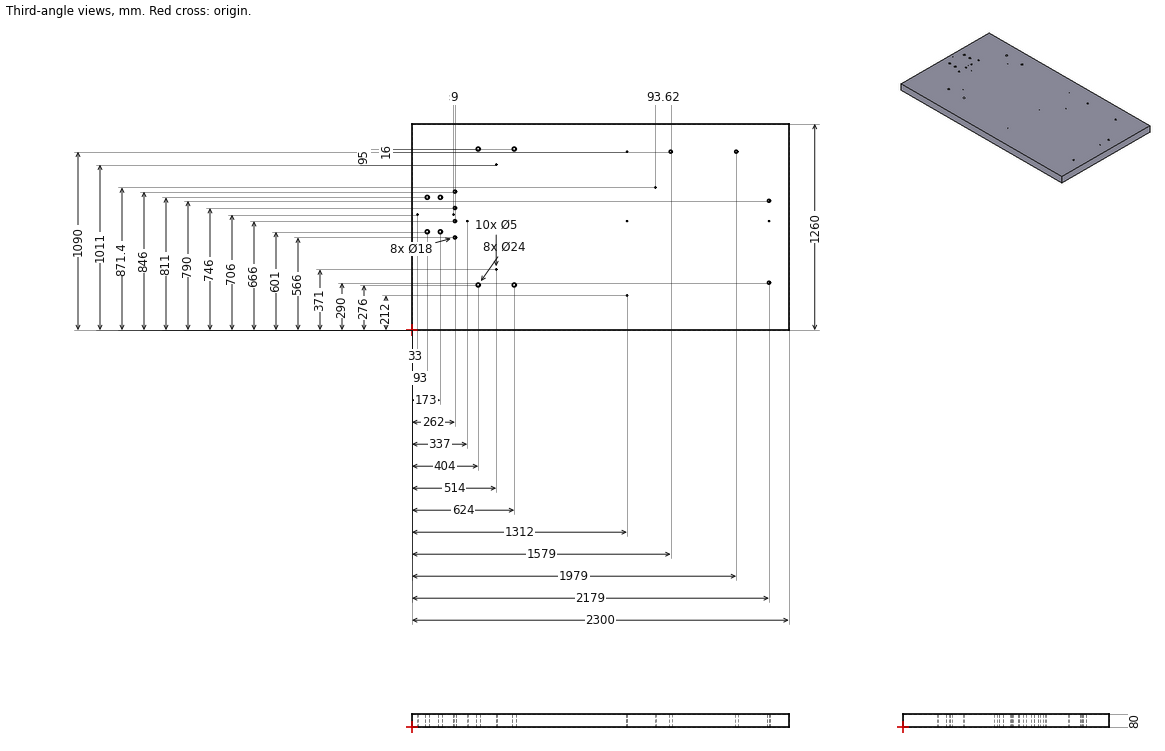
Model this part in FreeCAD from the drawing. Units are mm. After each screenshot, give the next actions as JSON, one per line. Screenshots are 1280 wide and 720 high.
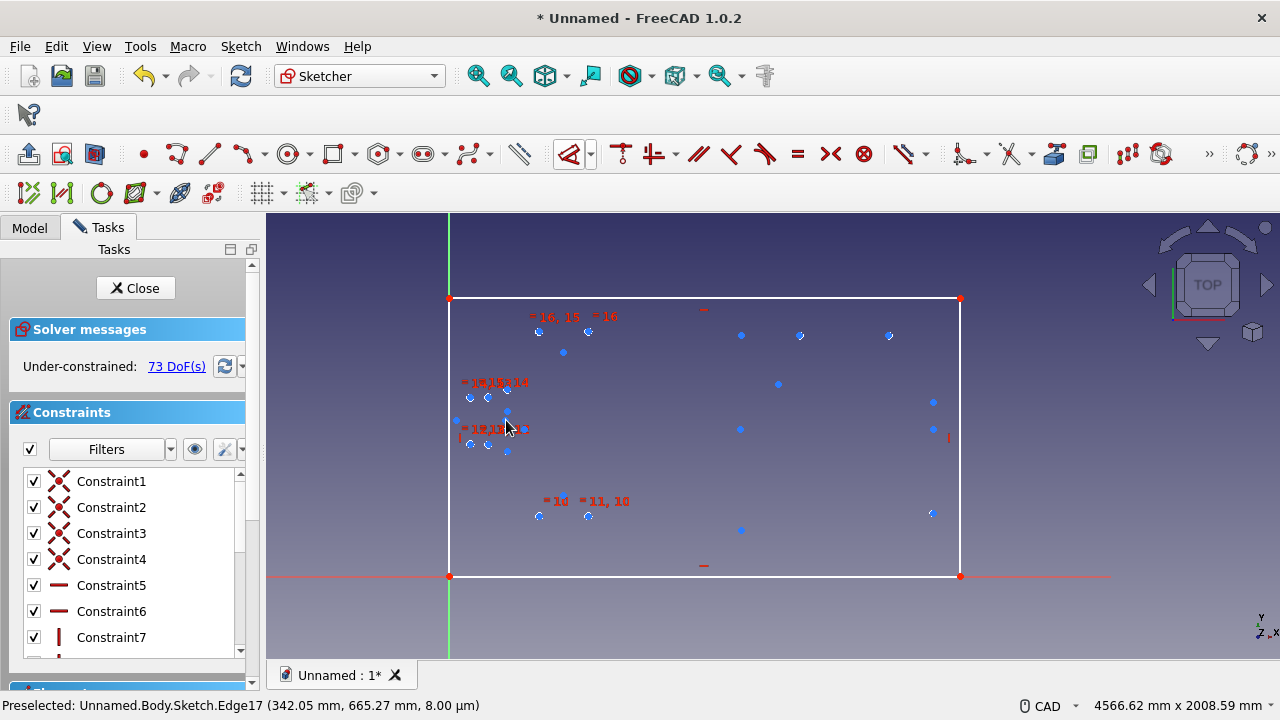
{"action": "scroll", "coordinate": [564, 352], "scroll_direction": "up", "scroll_amount": 12}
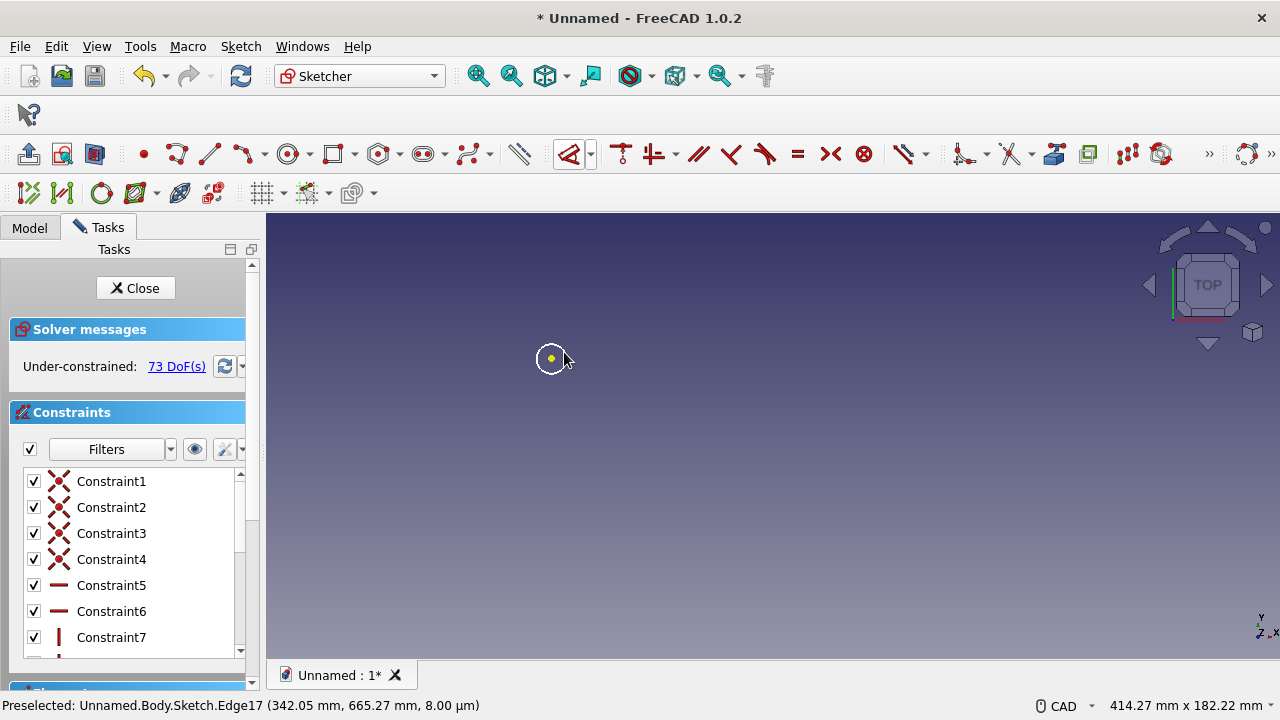
{"action": "left_click", "coordinate": [562, 349]}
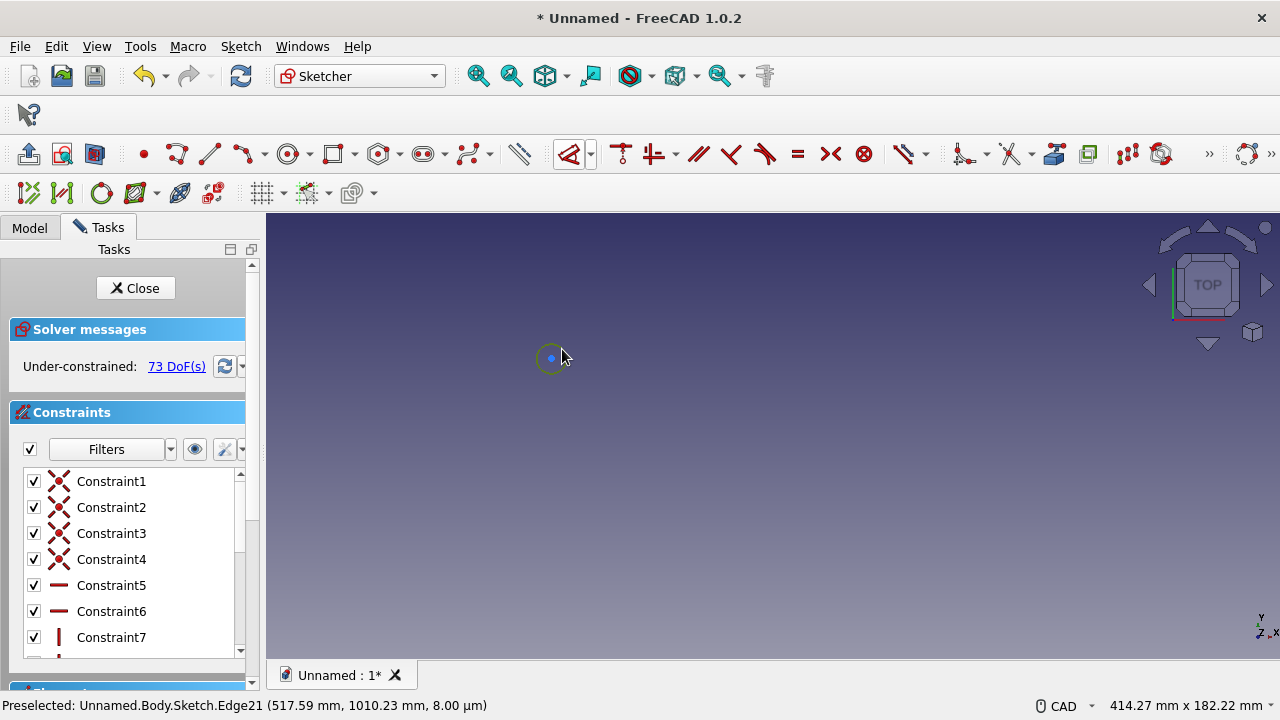
{"action": "scroll", "coordinate": [564, 351], "scroll_direction": "down", "scroll_amount": 12}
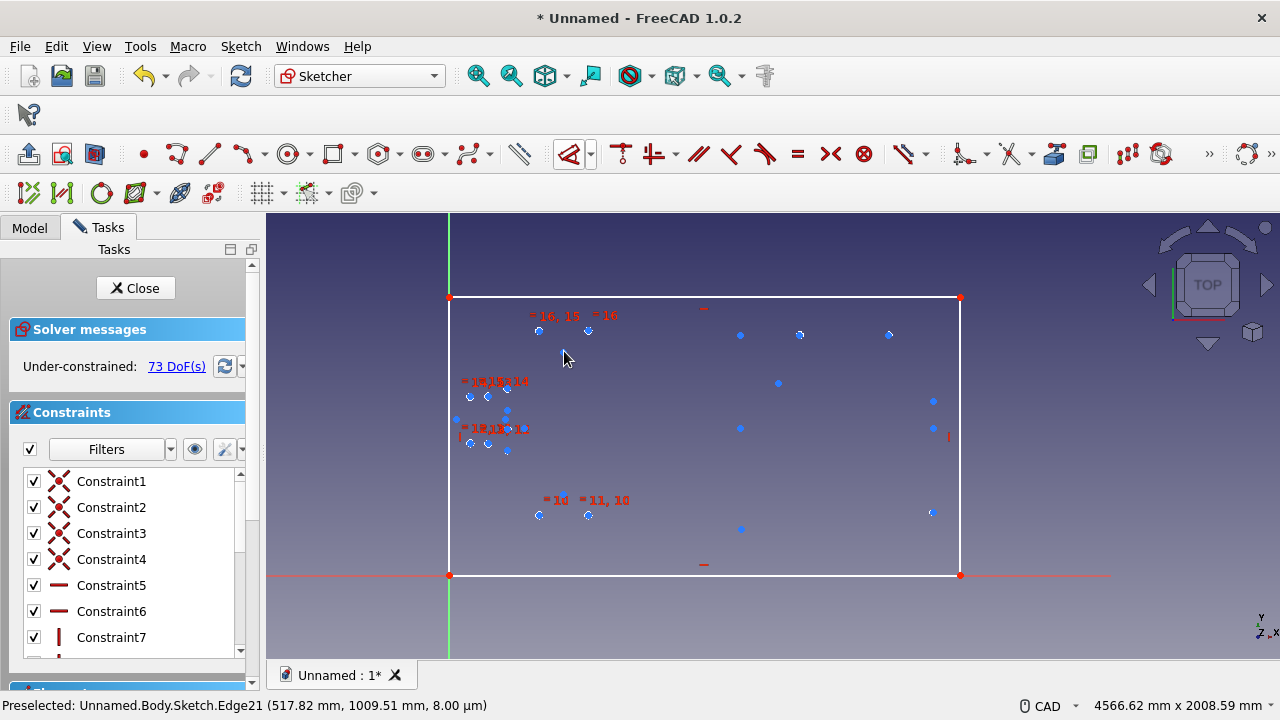
{"action": "scroll", "coordinate": [742, 428], "scroll_direction": "up", "scroll_amount": 13}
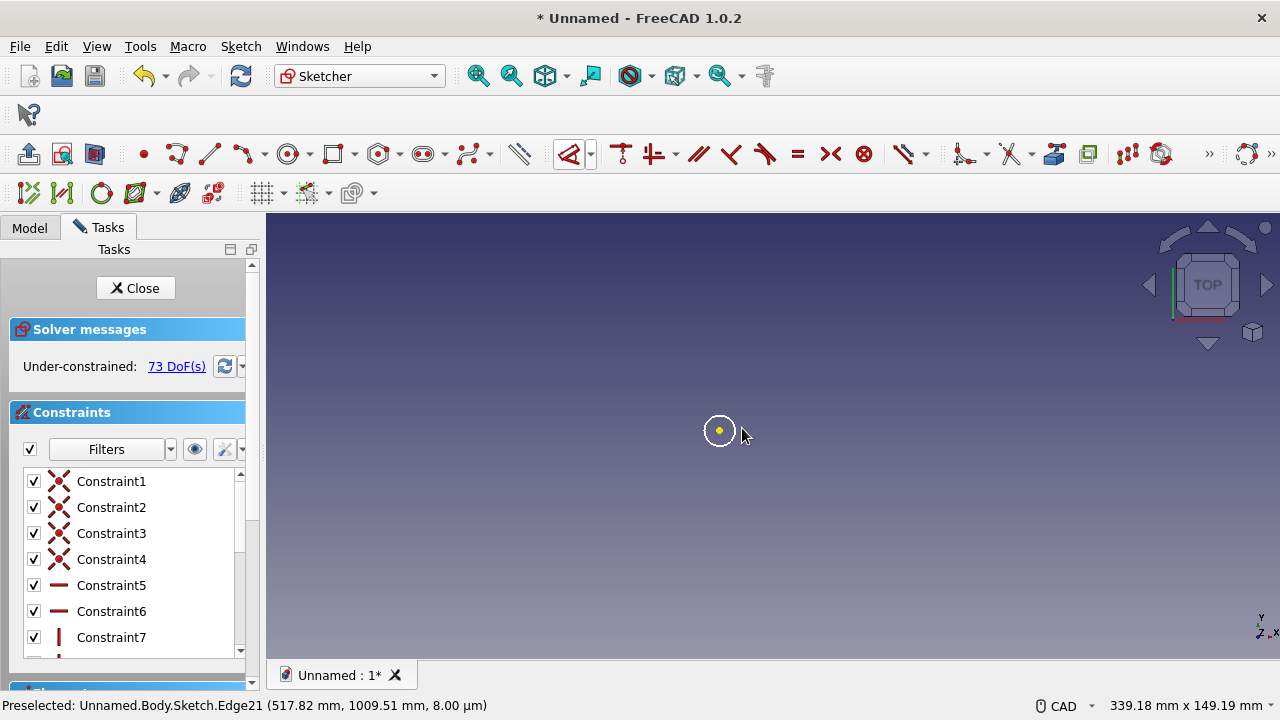
{"action": "left_click", "coordinate": [731, 420]}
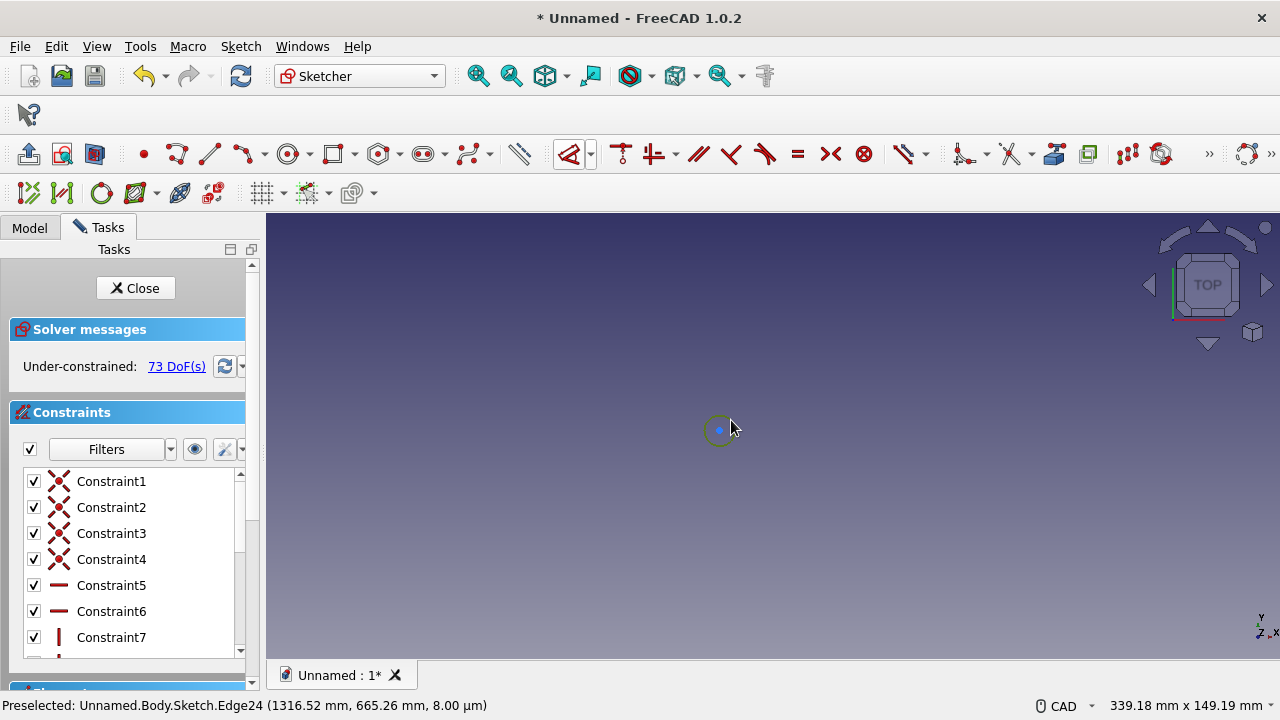
{"action": "scroll", "coordinate": [742, 429], "scroll_direction": "down", "scroll_amount": 13}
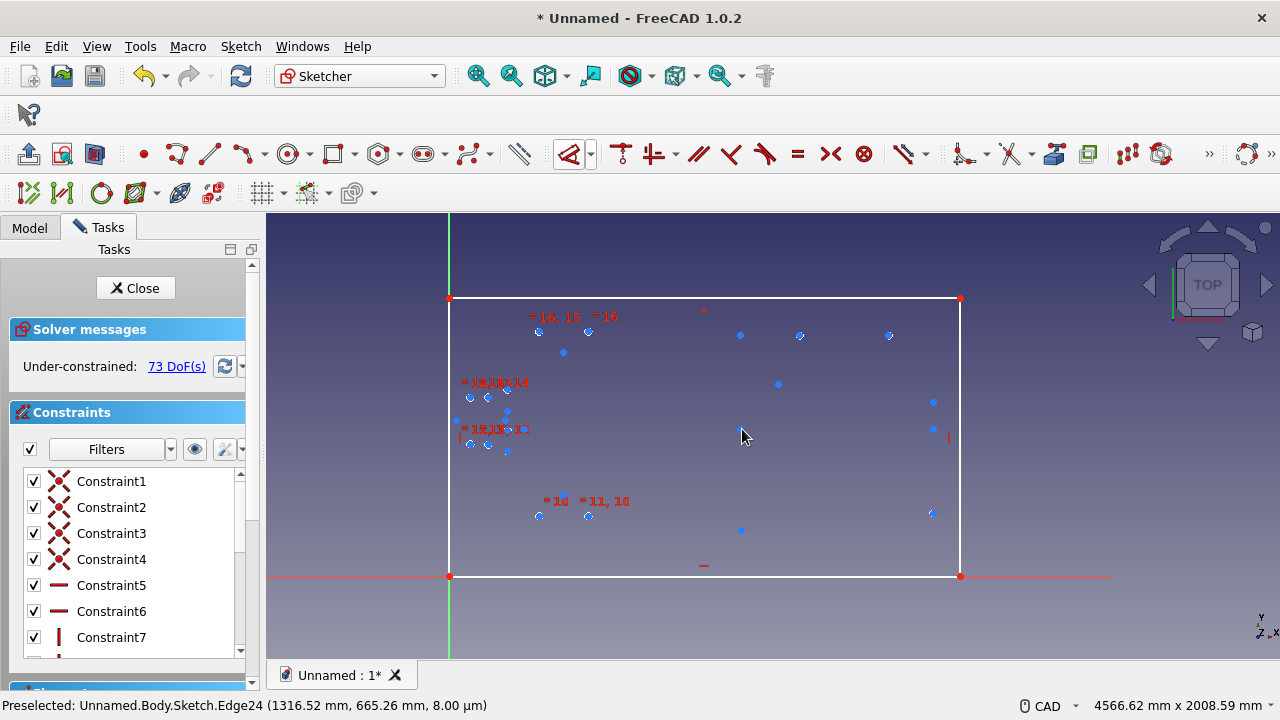
{"action": "scroll", "coordinate": [780, 383], "scroll_direction": "up", "scroll_amount": 11}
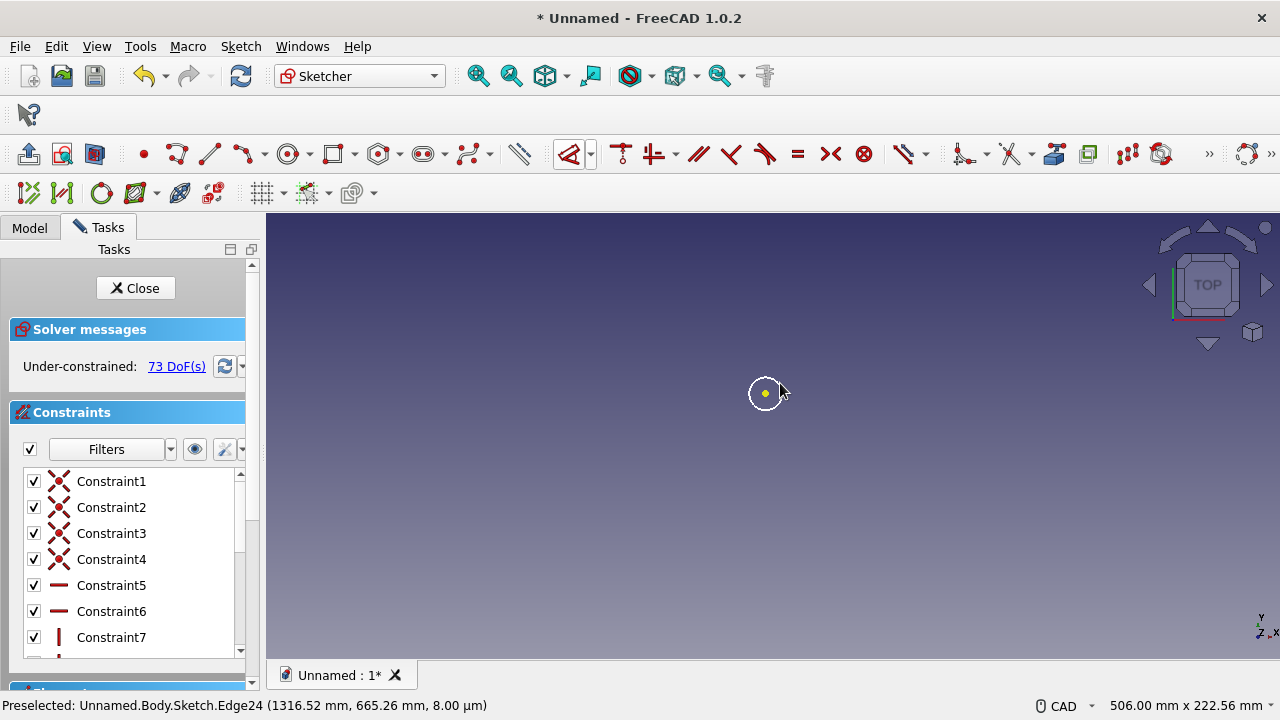
{"action": "left_click", "coordinate": [777, 382]}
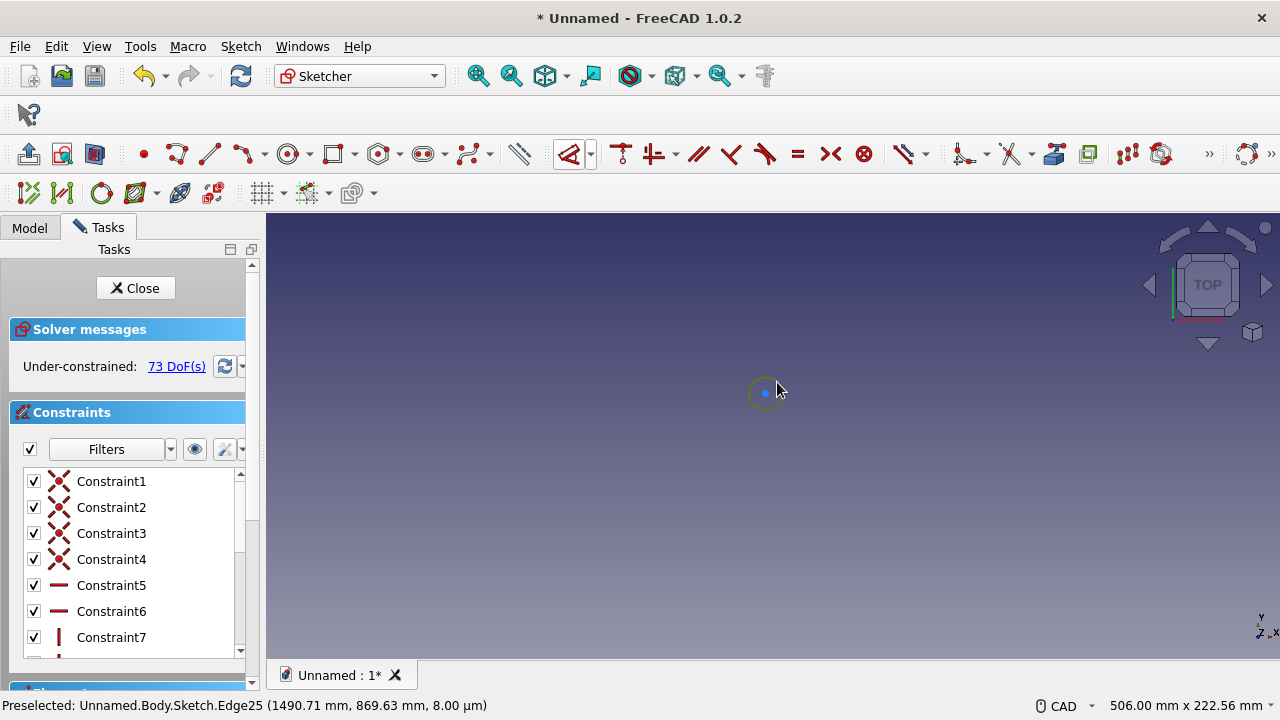
{"action": "scroll", "coordinate": [780, 382], "scroll_direction": "down", "scroll_amount": 11}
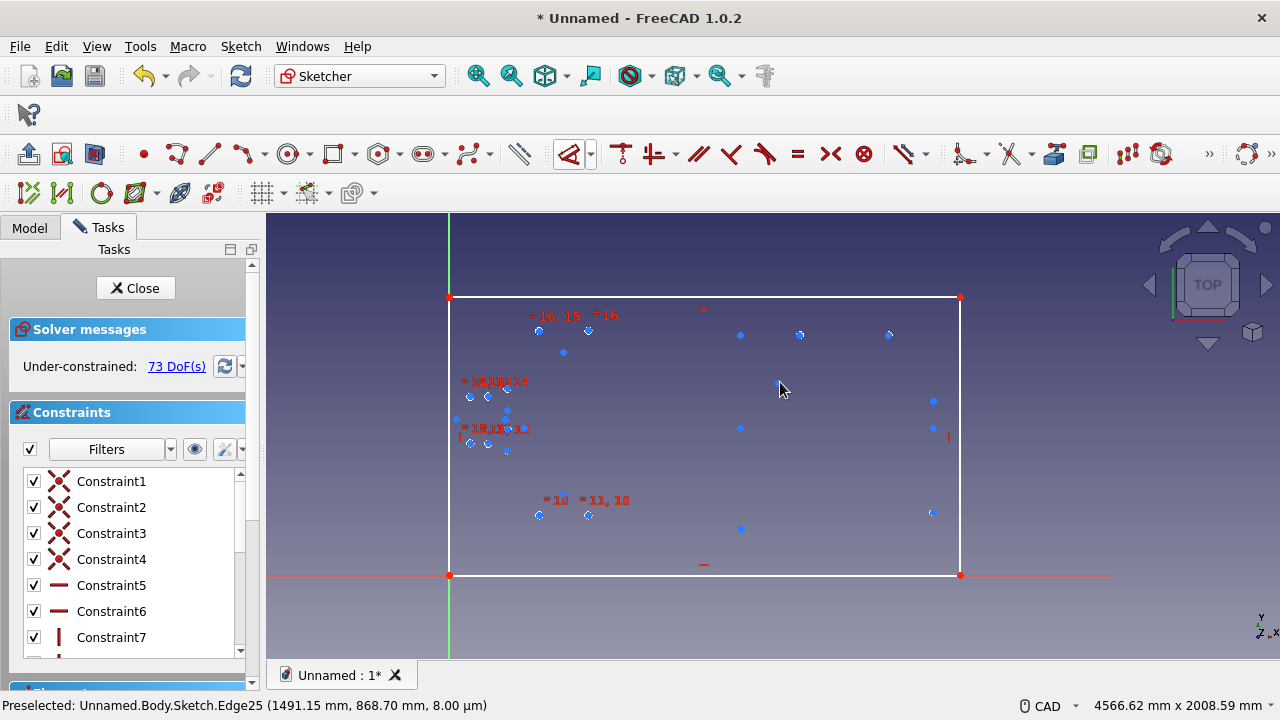
{"action": "scroll", "coordinate": [933, 429], "scroll_direction": "up", "scroll_amount": 14}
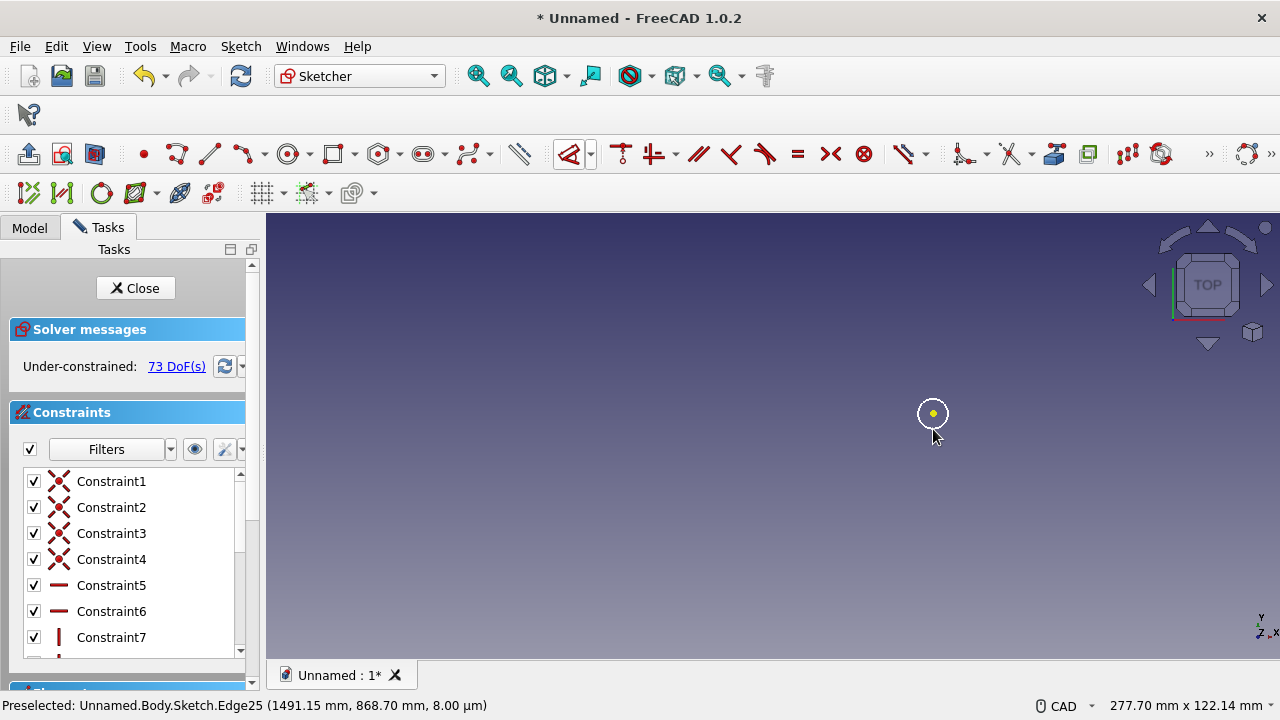
{"action": "left_click", "coordinate": [918, 413]}